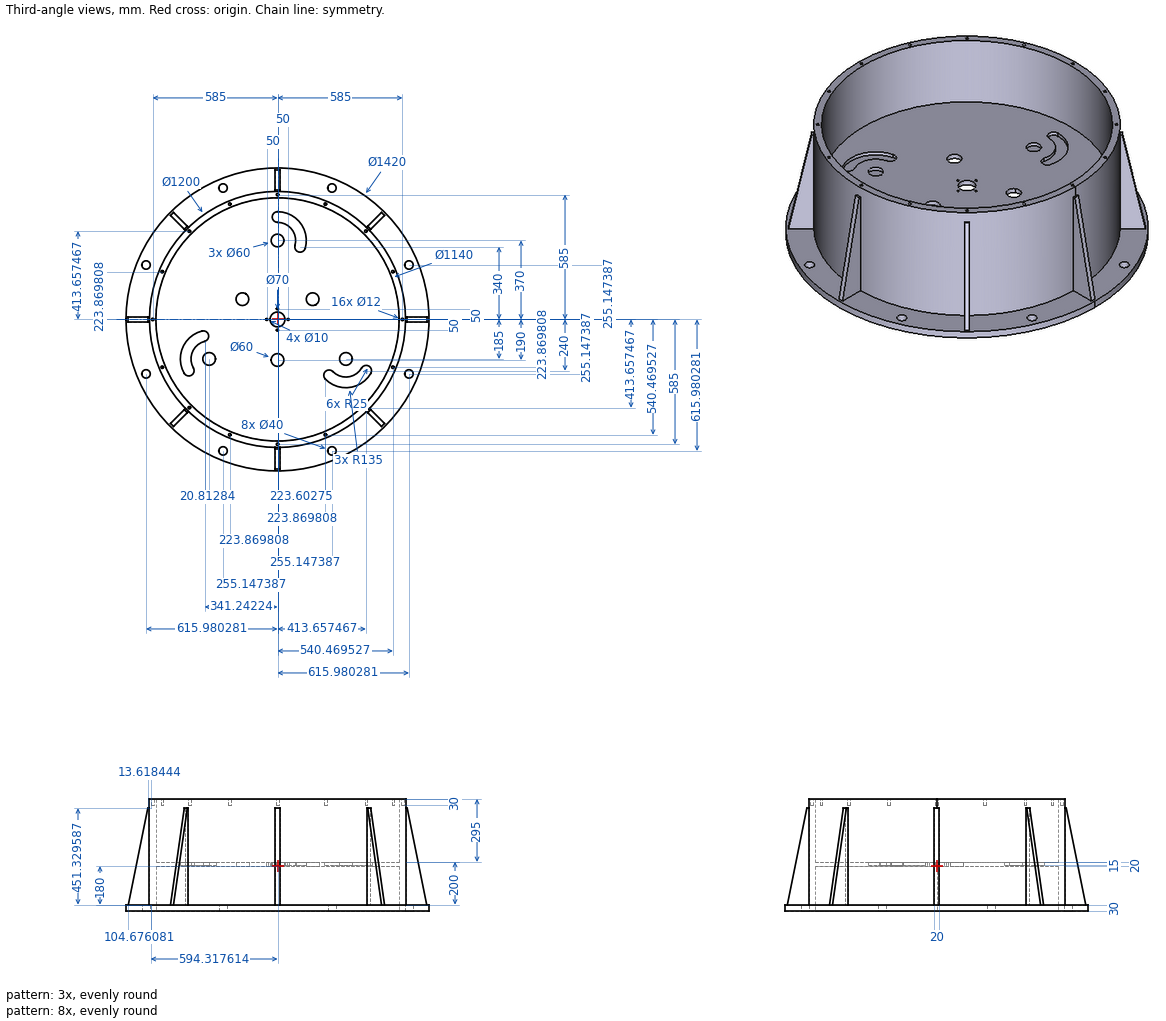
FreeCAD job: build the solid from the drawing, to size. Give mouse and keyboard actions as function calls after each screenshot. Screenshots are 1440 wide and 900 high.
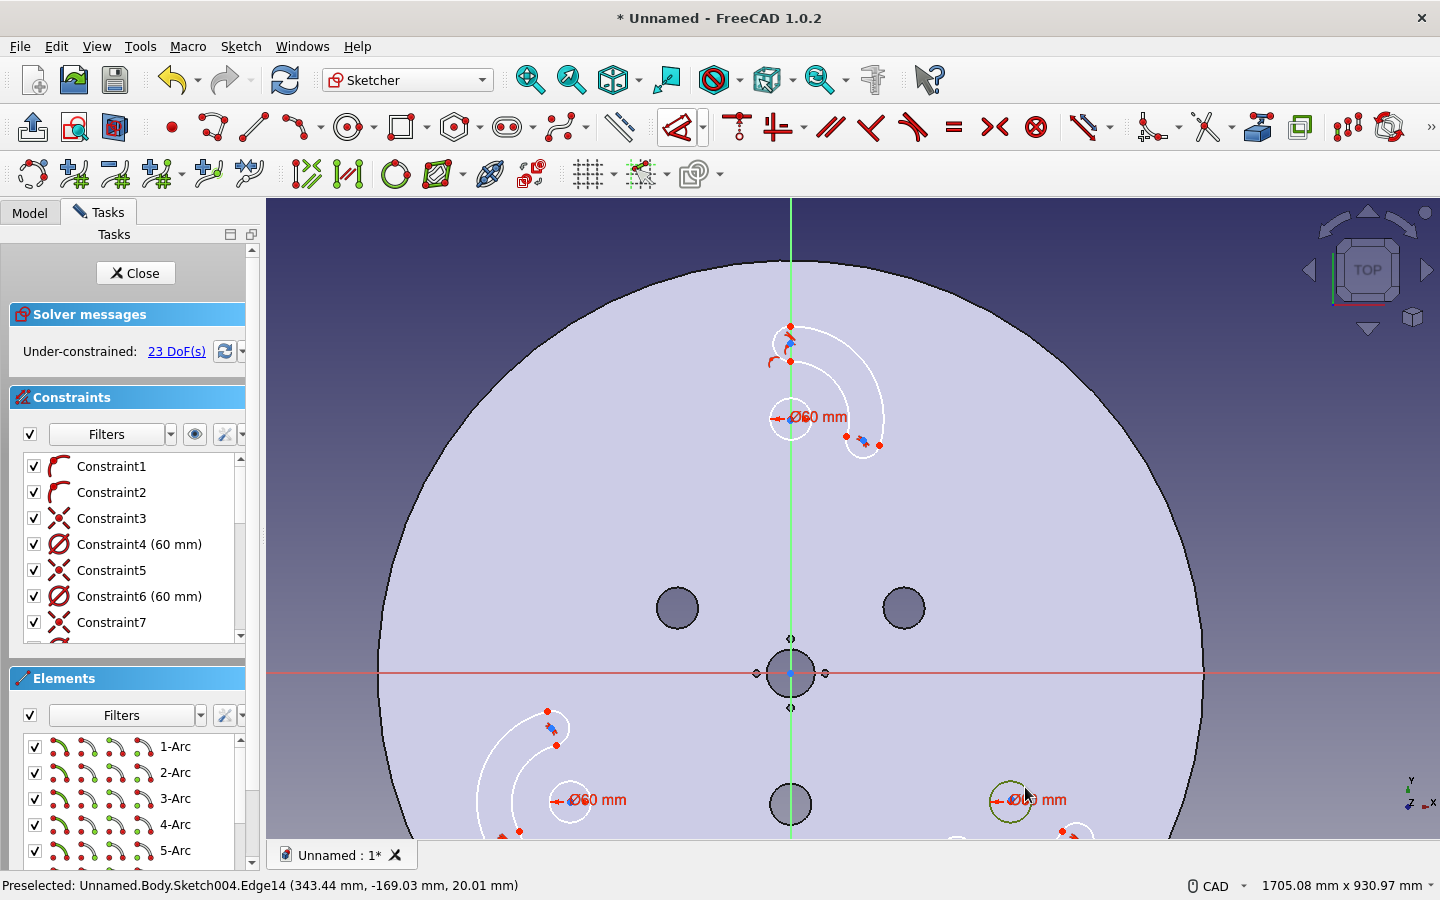
scroll(777, 334, down, 2)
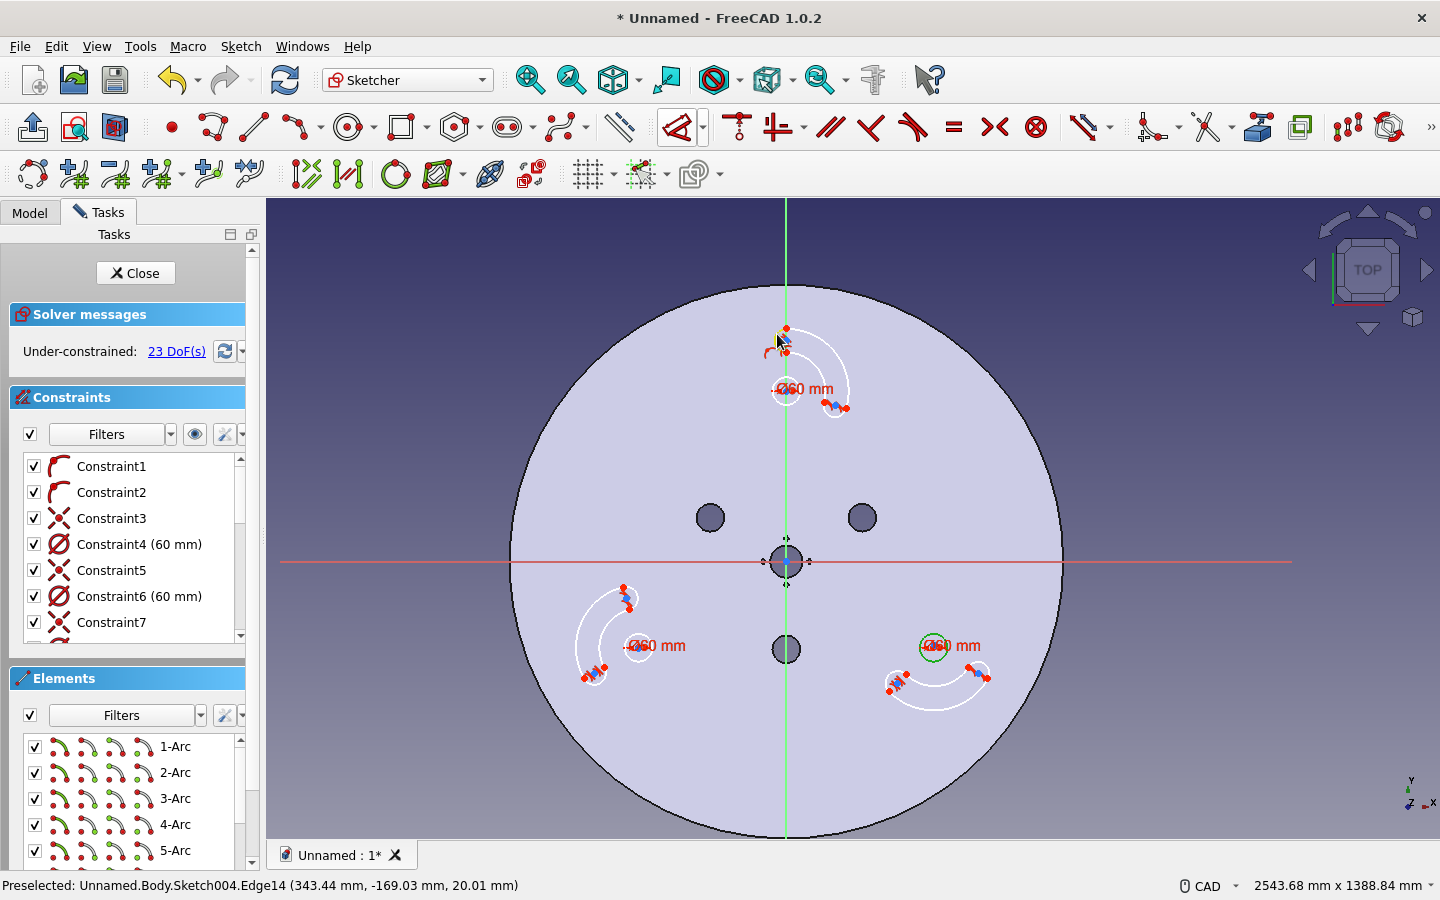
click(925, 685)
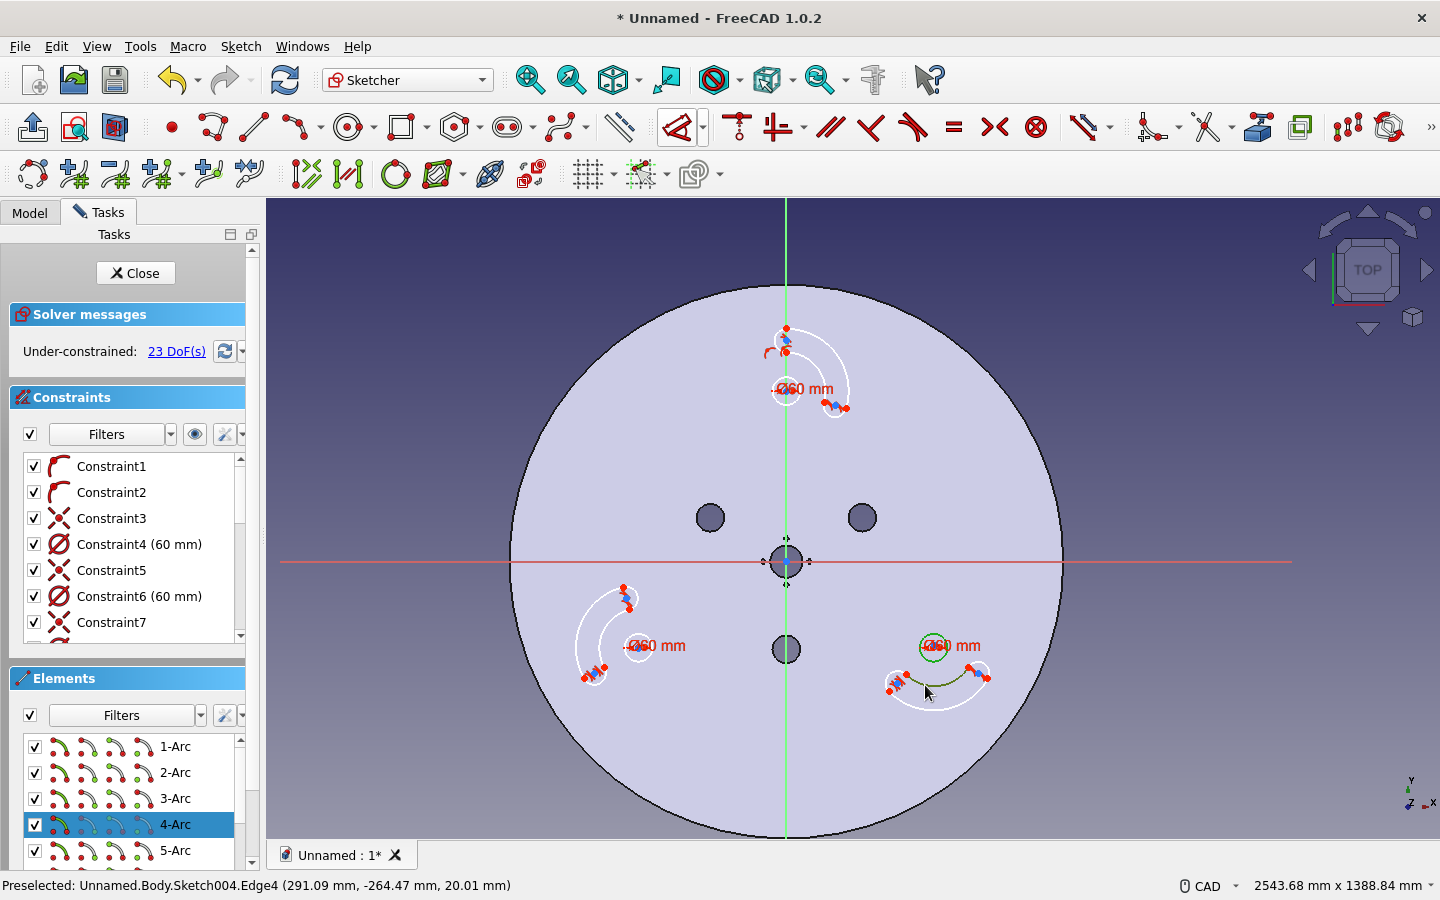
key(c)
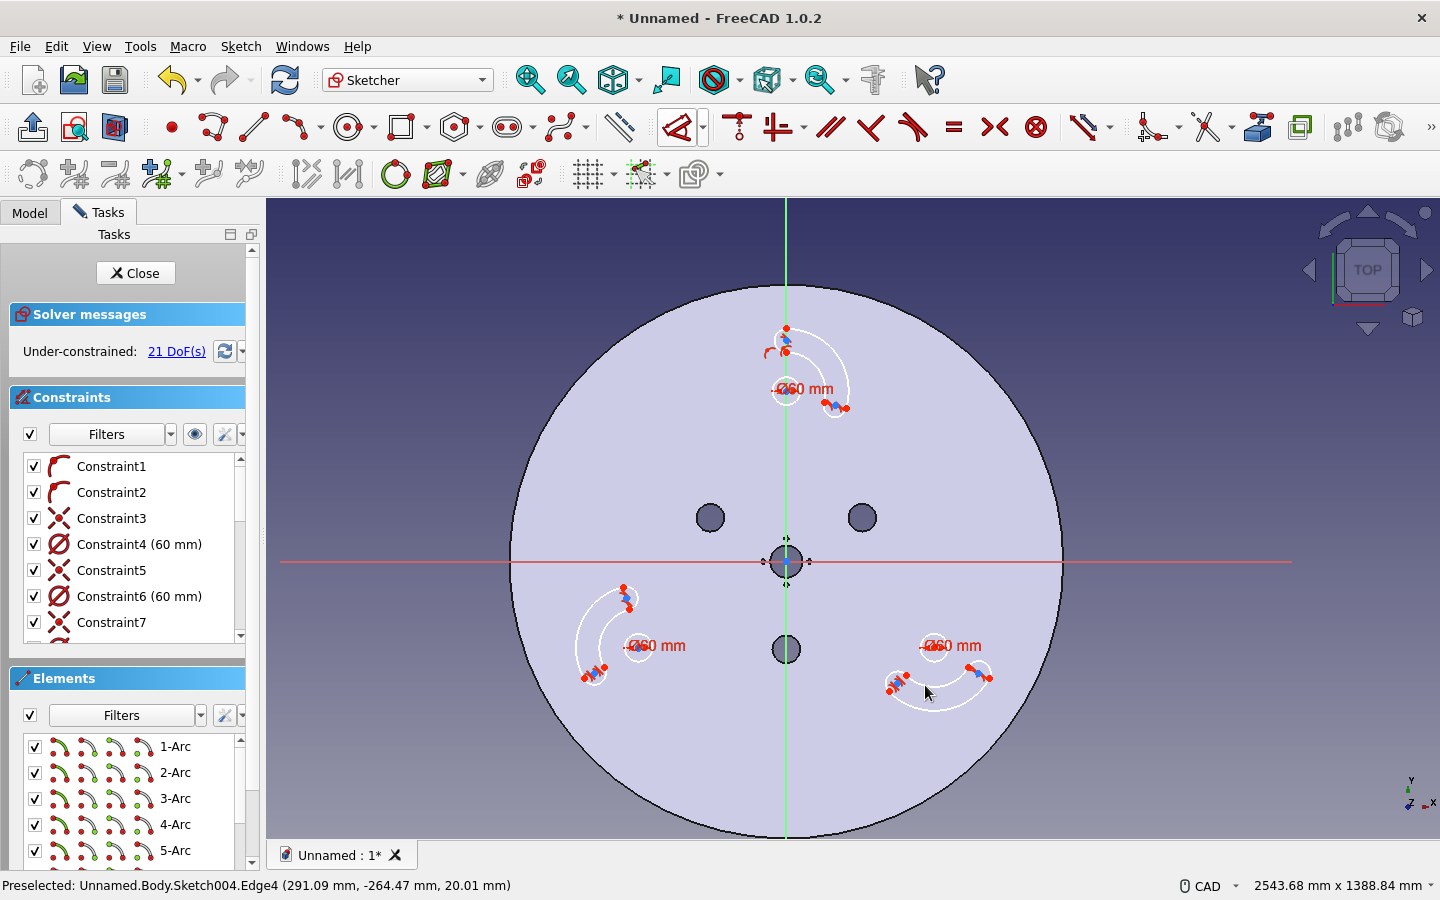
click(648, 638)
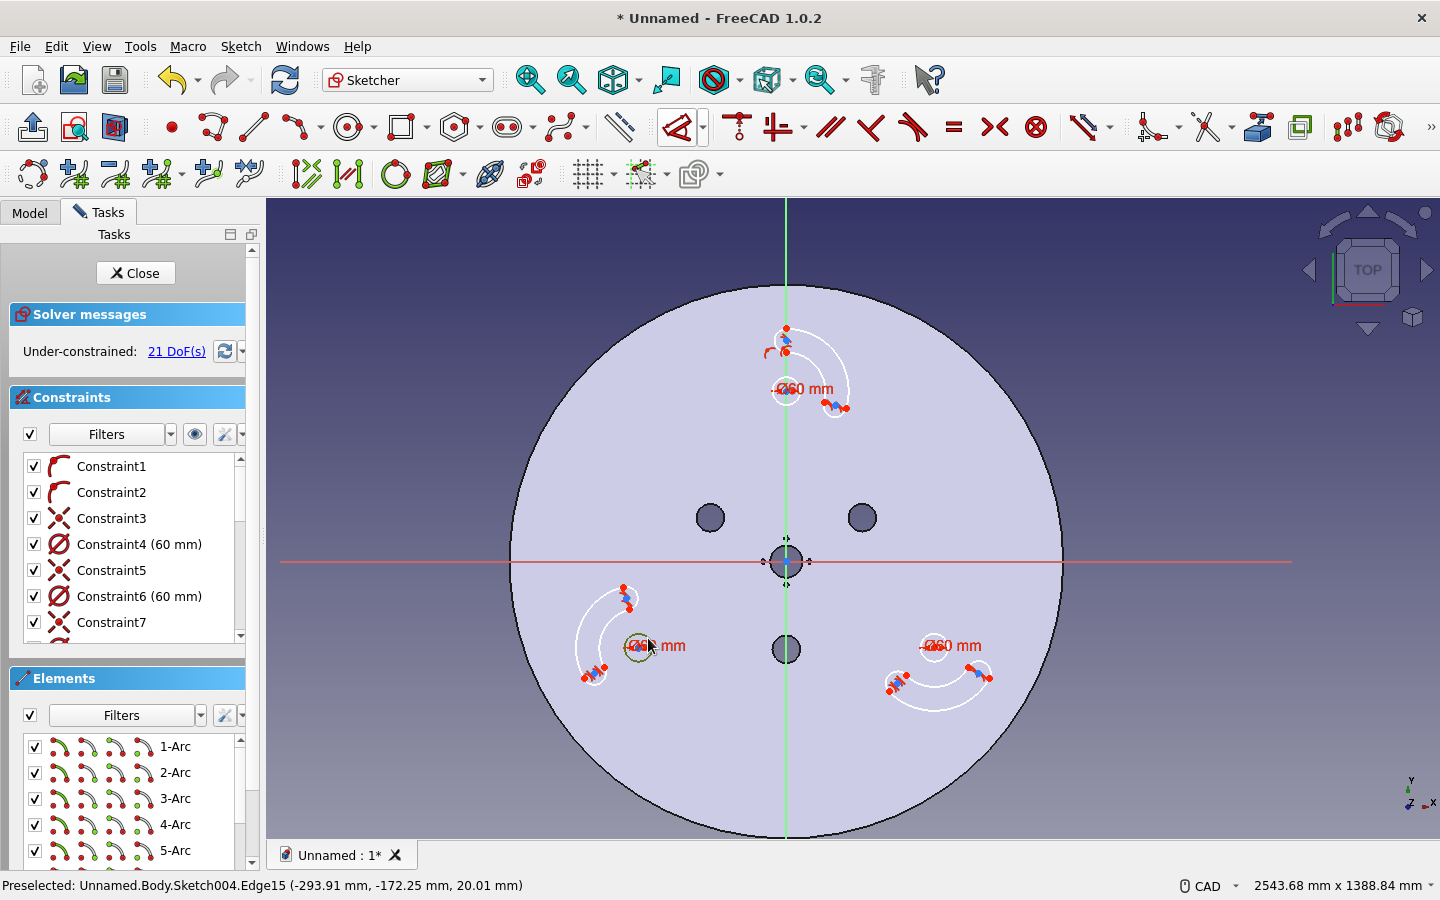
click(611, 621)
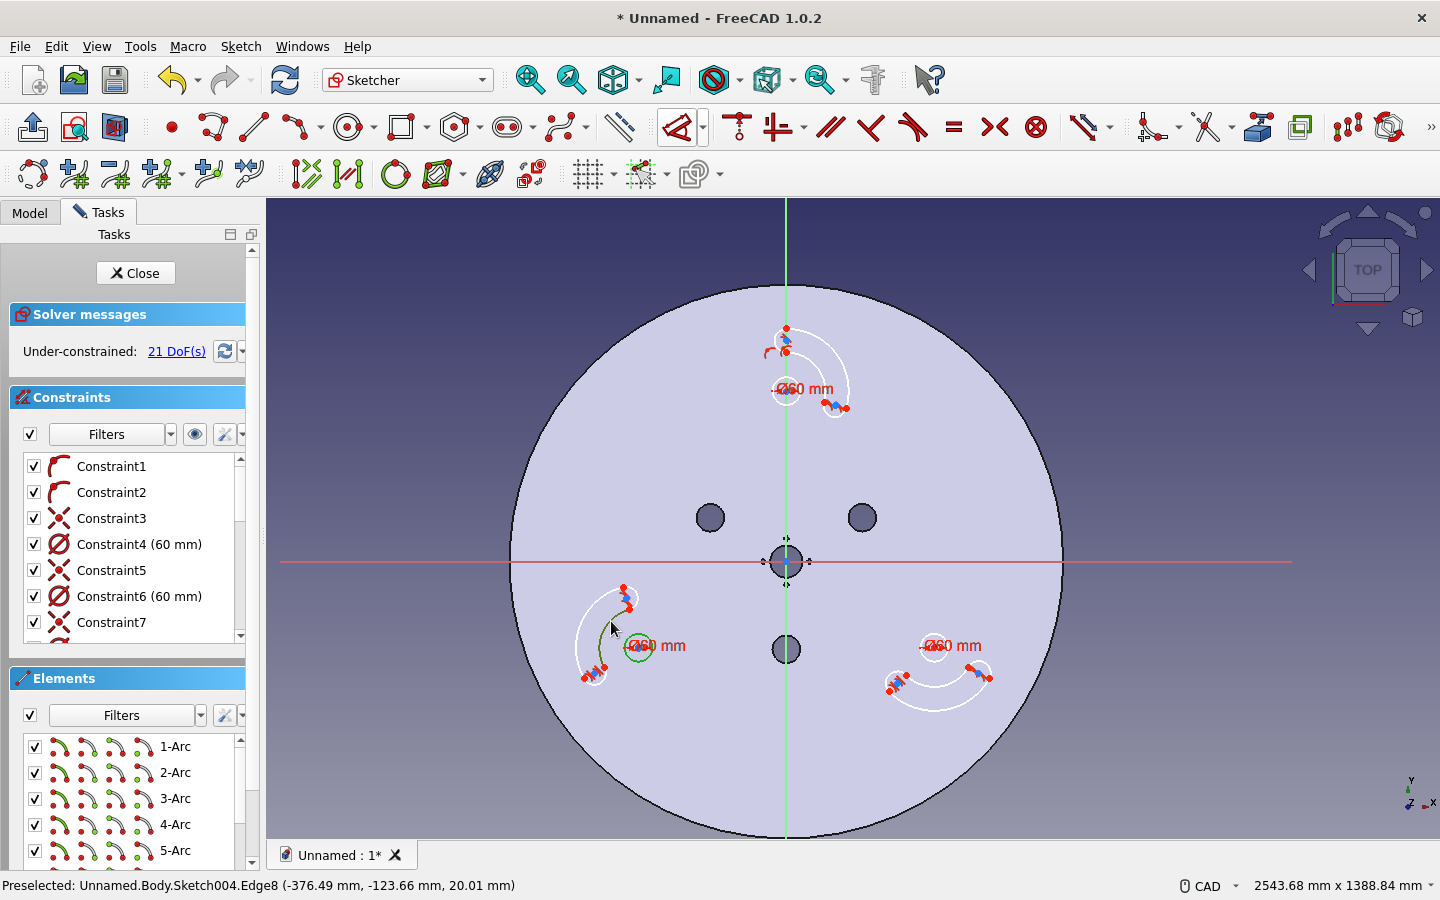
click(737, 128)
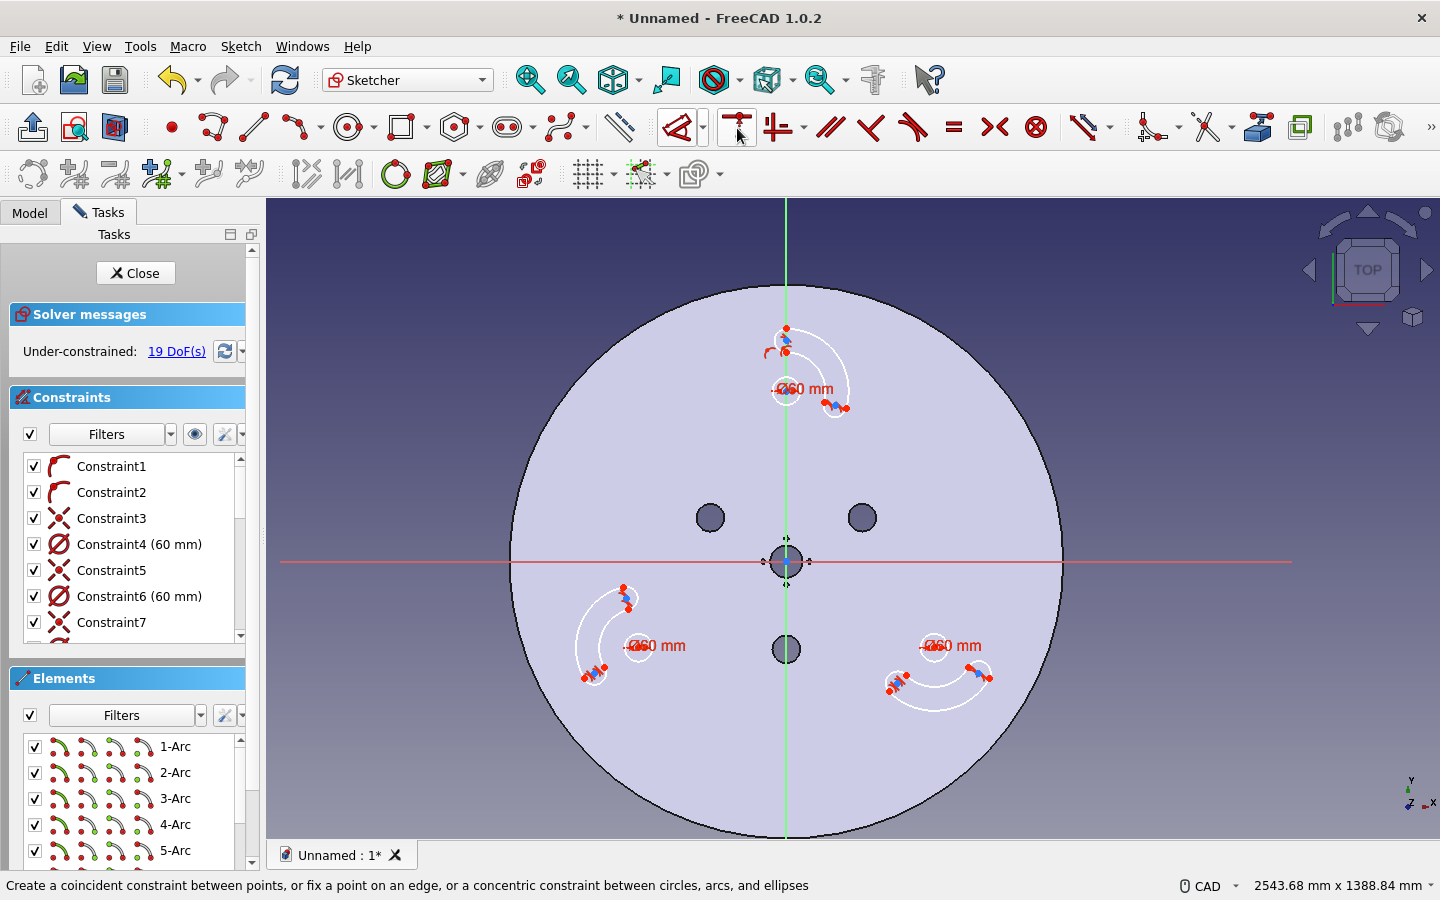
scroll(796, 381, up, 2)